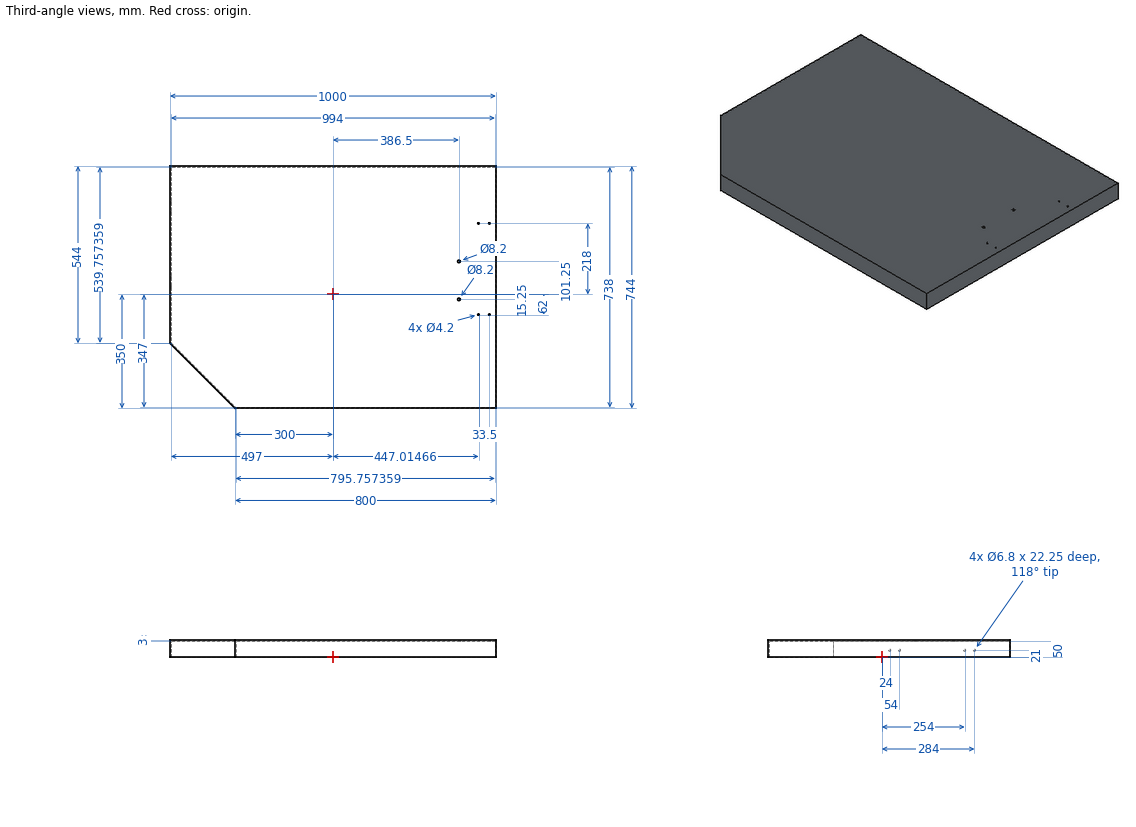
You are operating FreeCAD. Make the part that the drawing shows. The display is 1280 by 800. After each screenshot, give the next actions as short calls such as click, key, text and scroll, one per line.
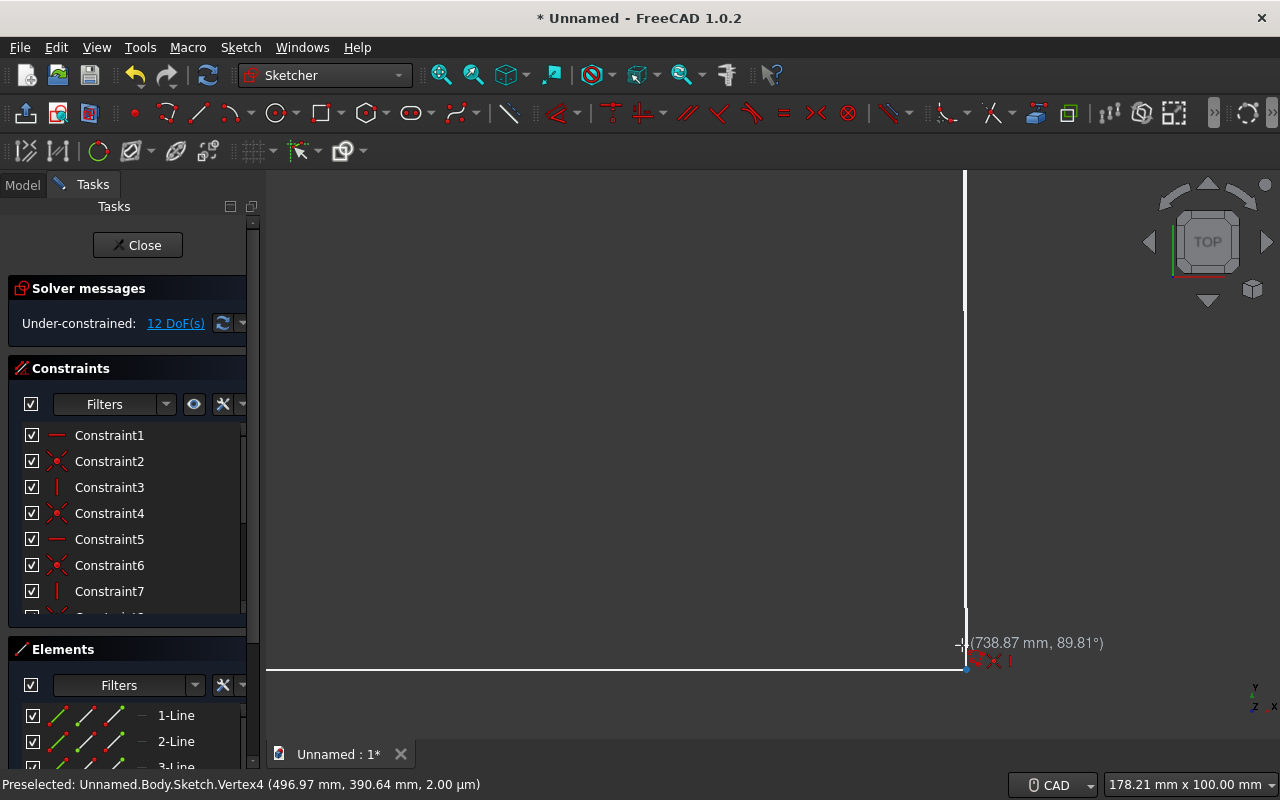
click(952, 642)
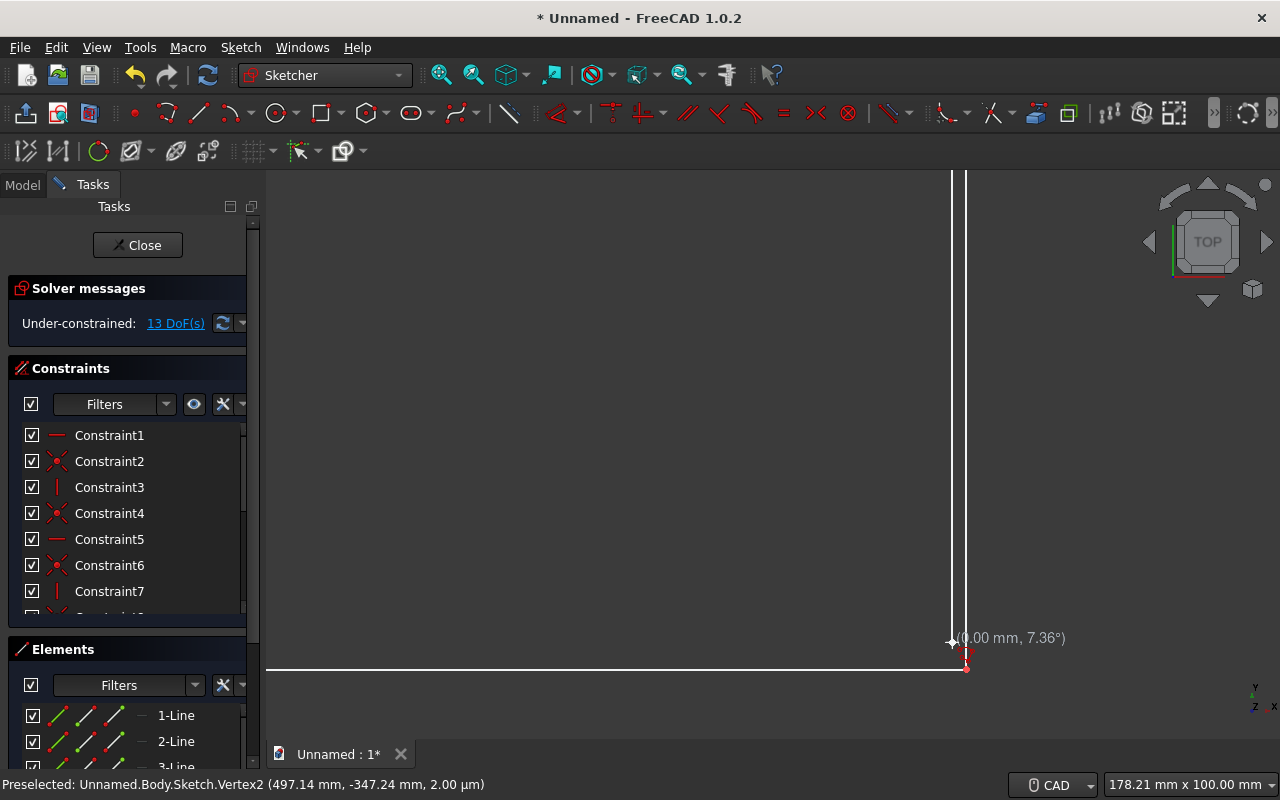
scroll(962, 645, down, 12)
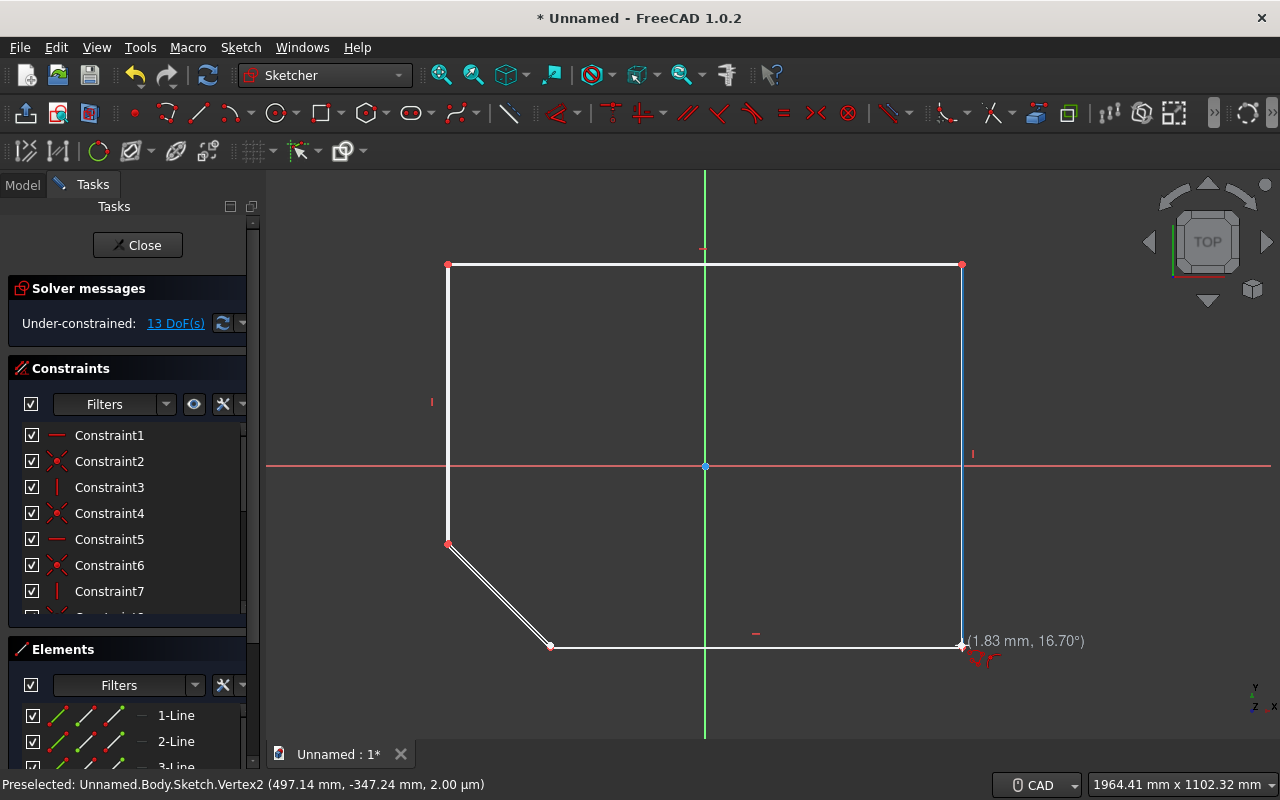
scroll(551, 645, up, 12)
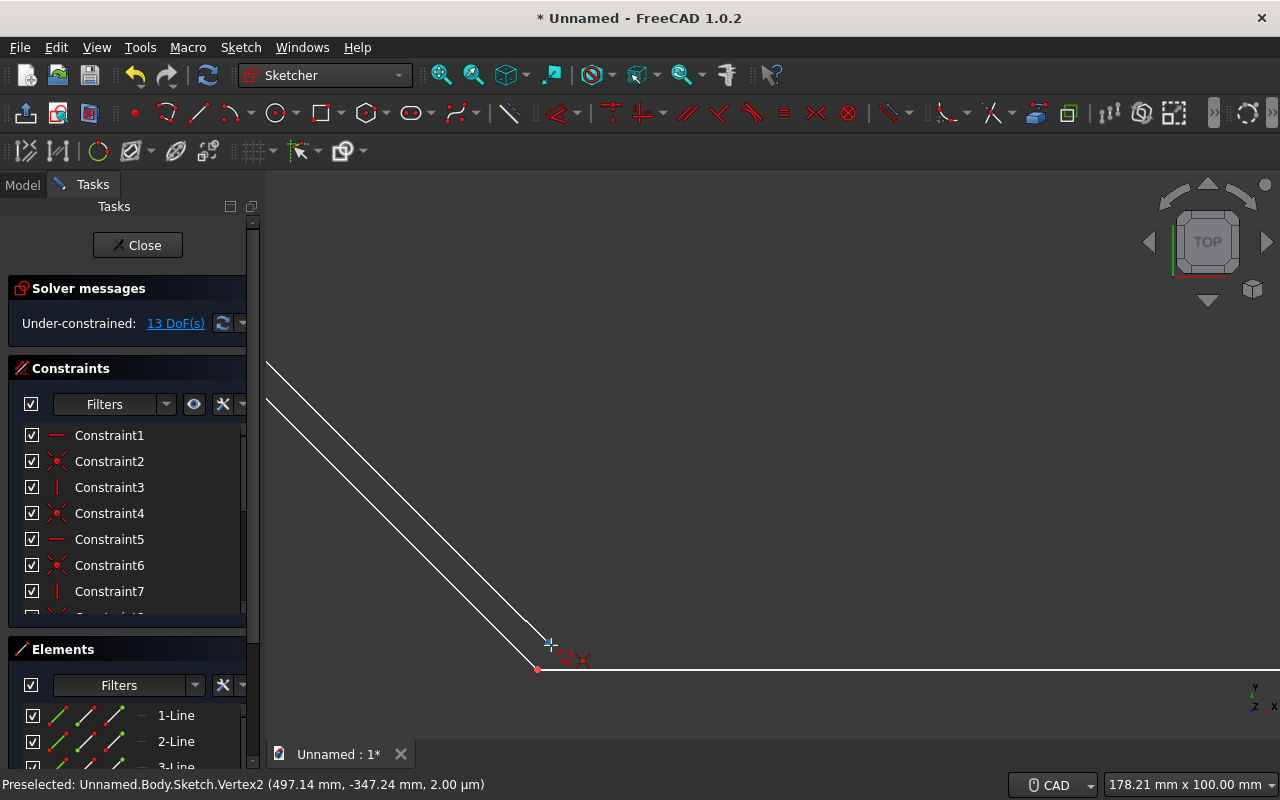
click(548, 643)
key(Escape)
key(Escape)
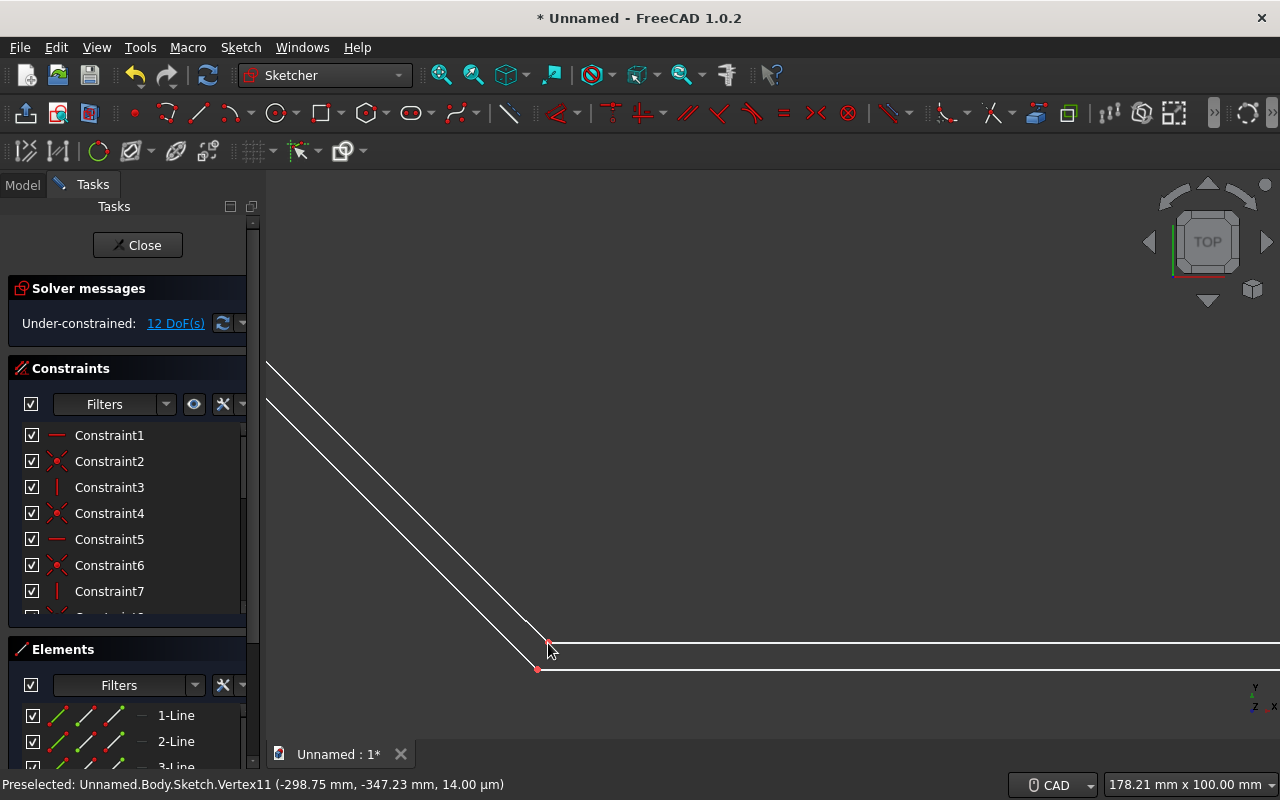
click(556, 114)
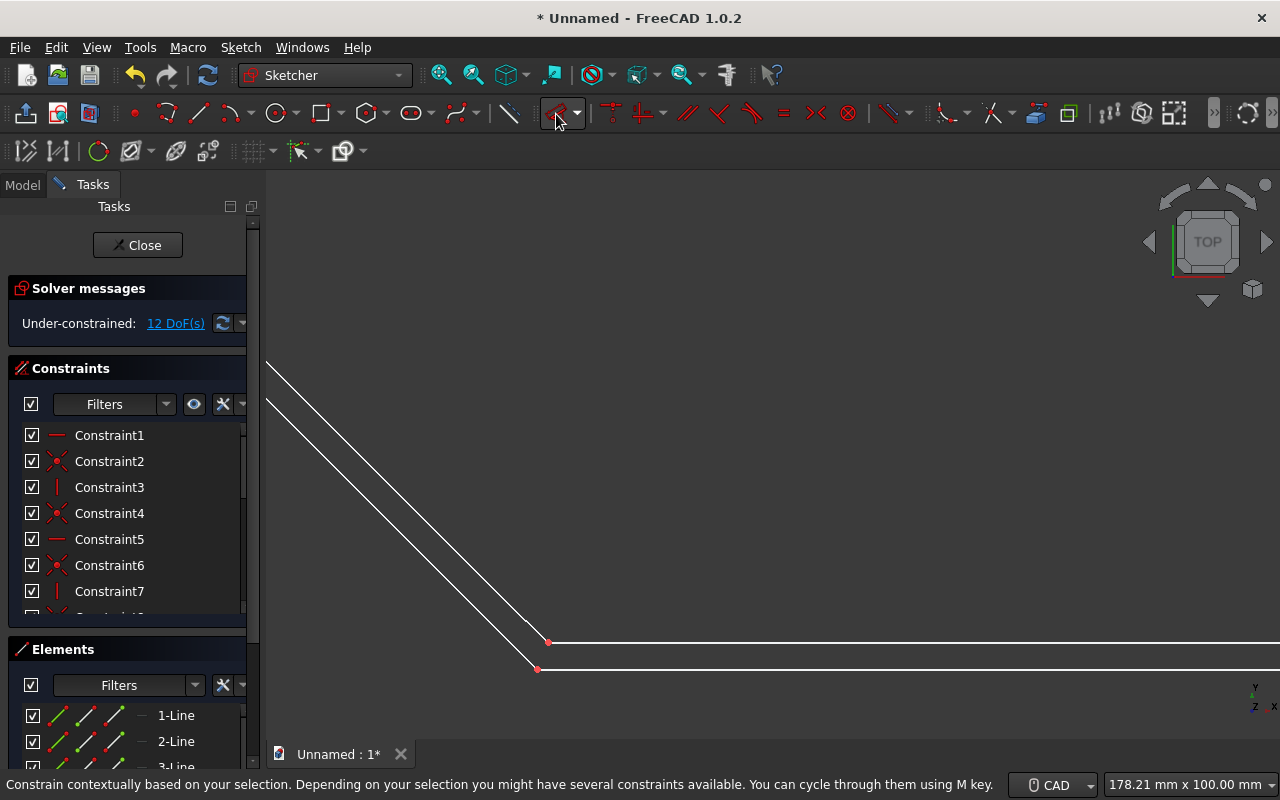
scroll(551, 645, down, 12)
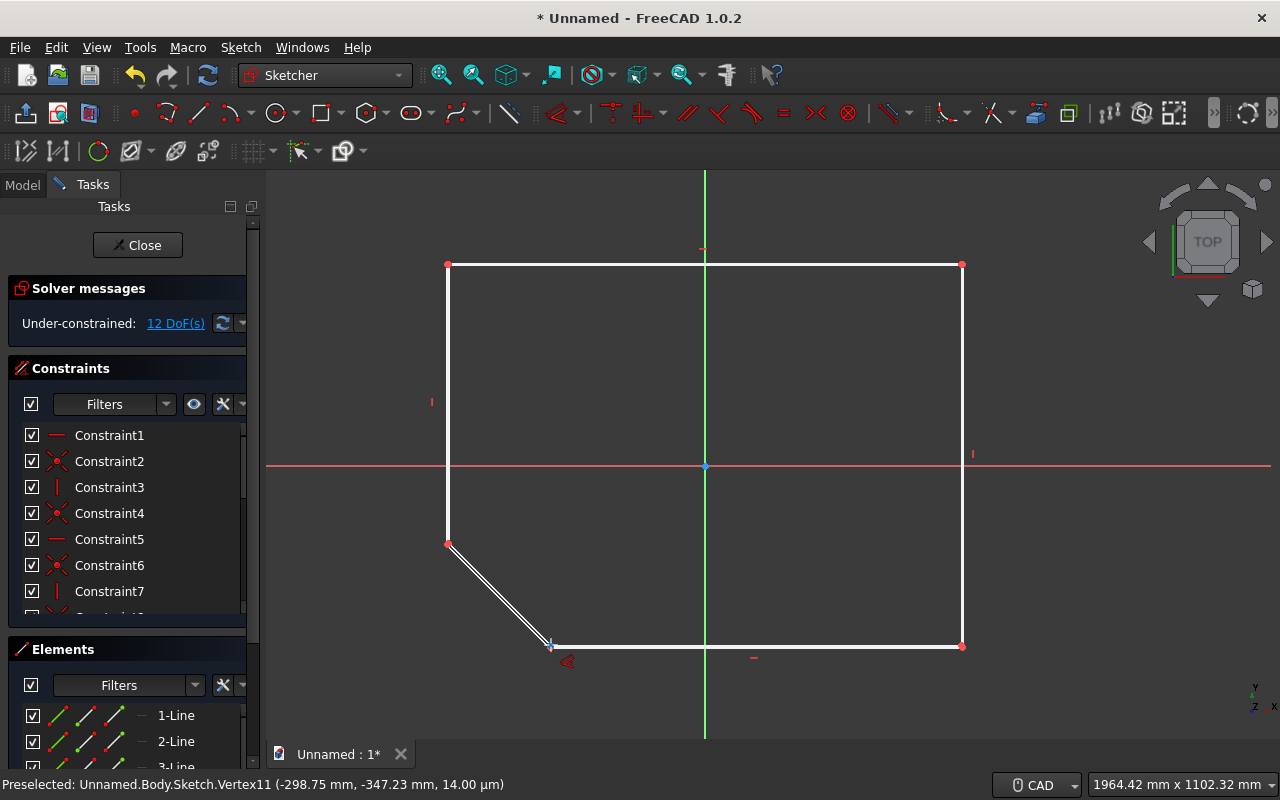
scroll(674, 648, up, 9)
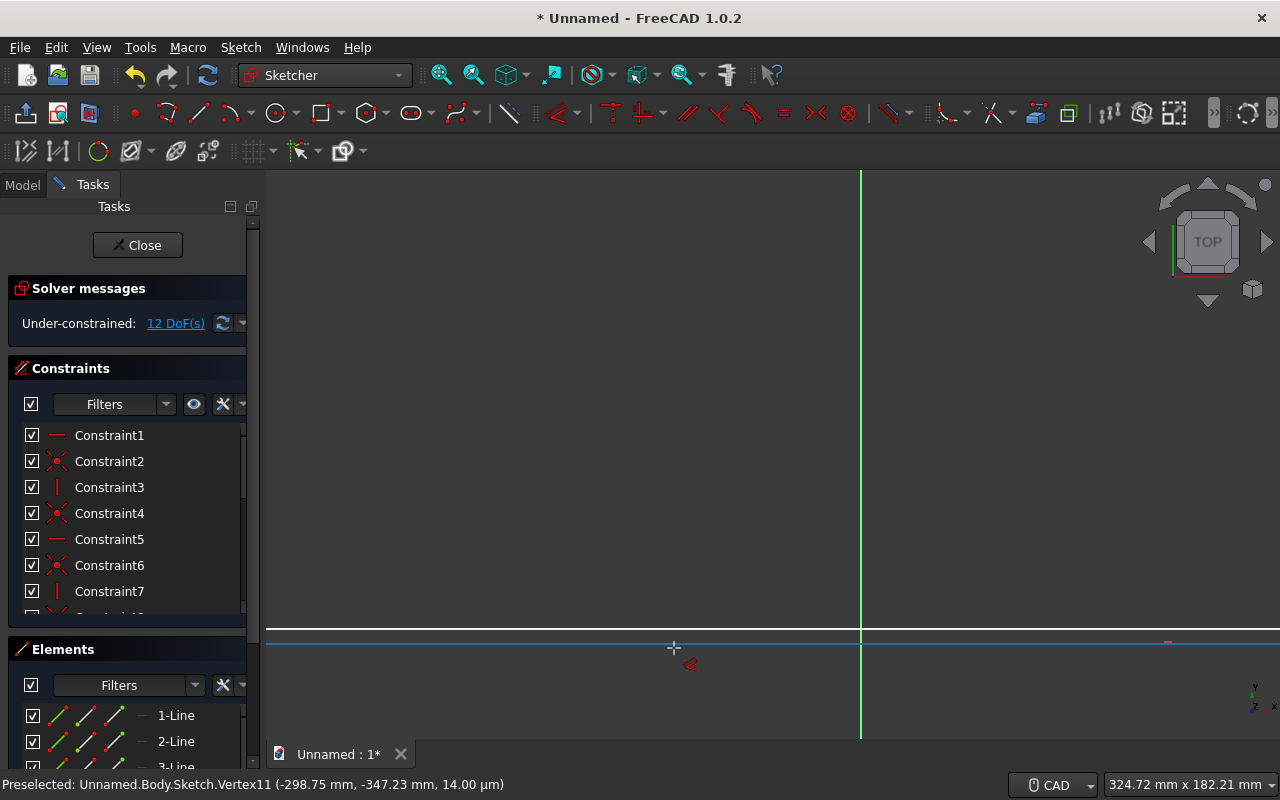
click(671, 644)
click(704, 678)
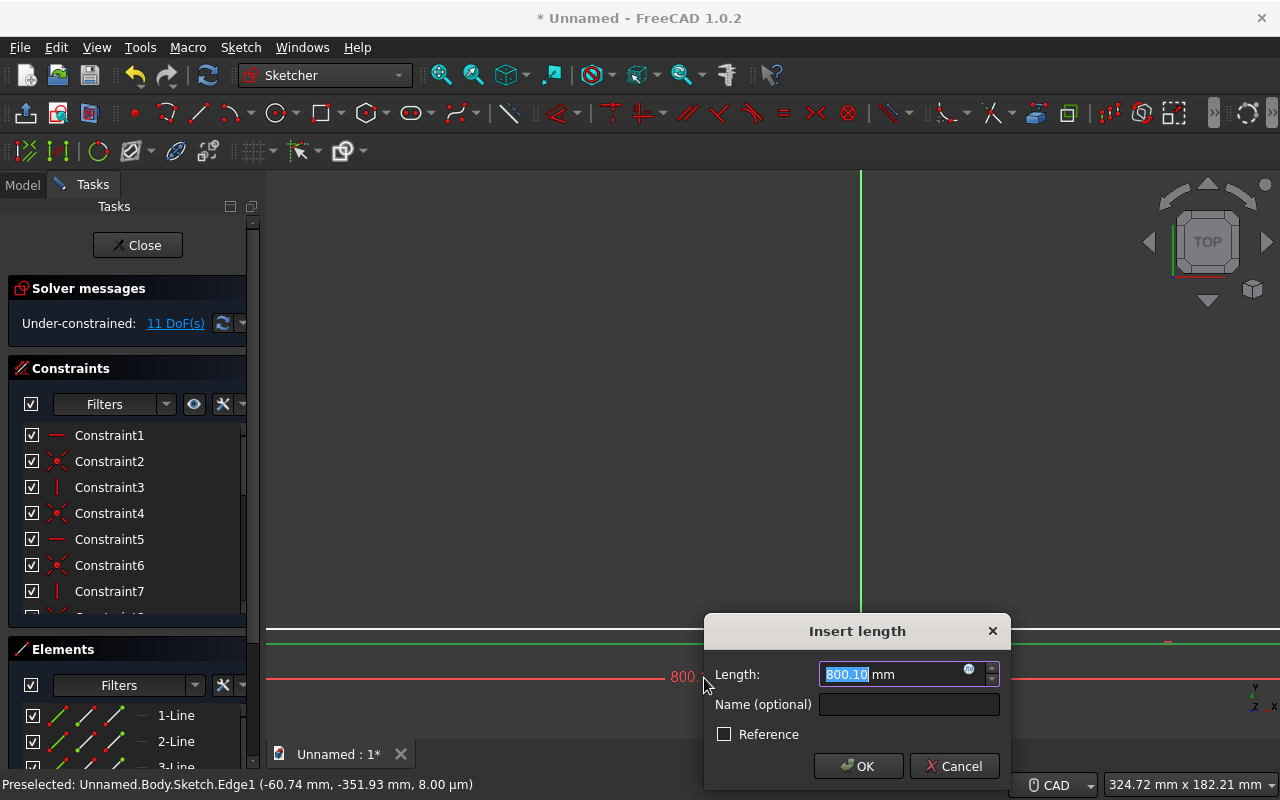
text(800)
key(Return)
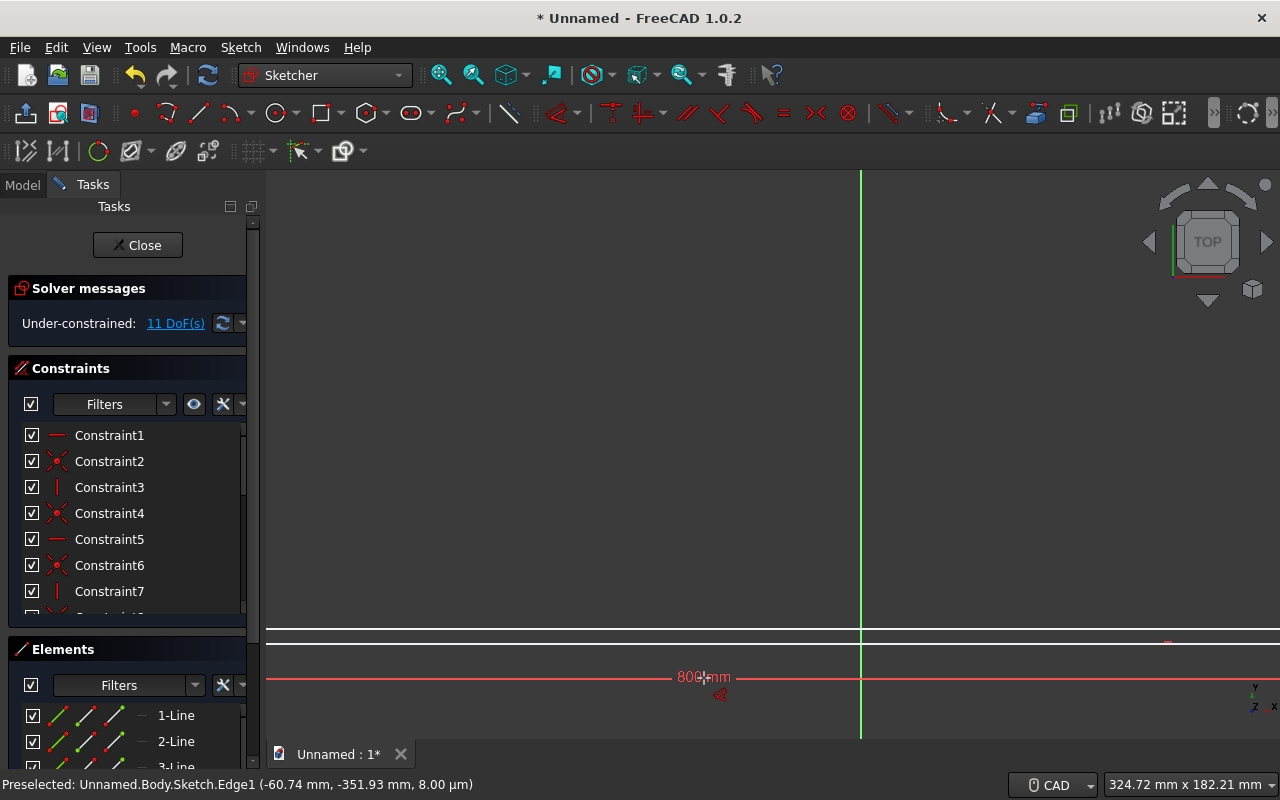
scroll(674, 648, down, 9)